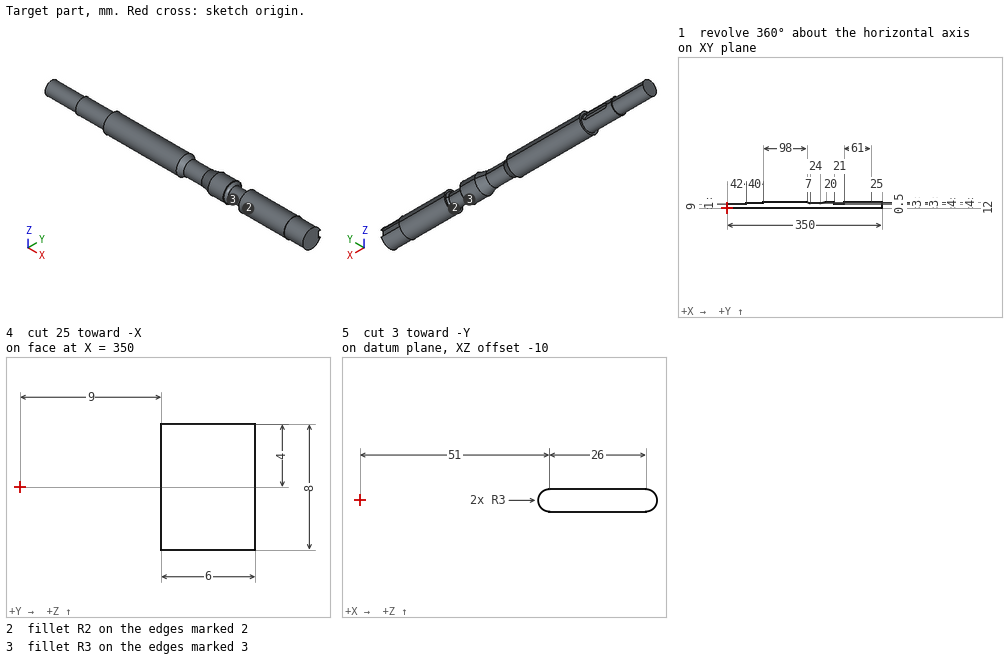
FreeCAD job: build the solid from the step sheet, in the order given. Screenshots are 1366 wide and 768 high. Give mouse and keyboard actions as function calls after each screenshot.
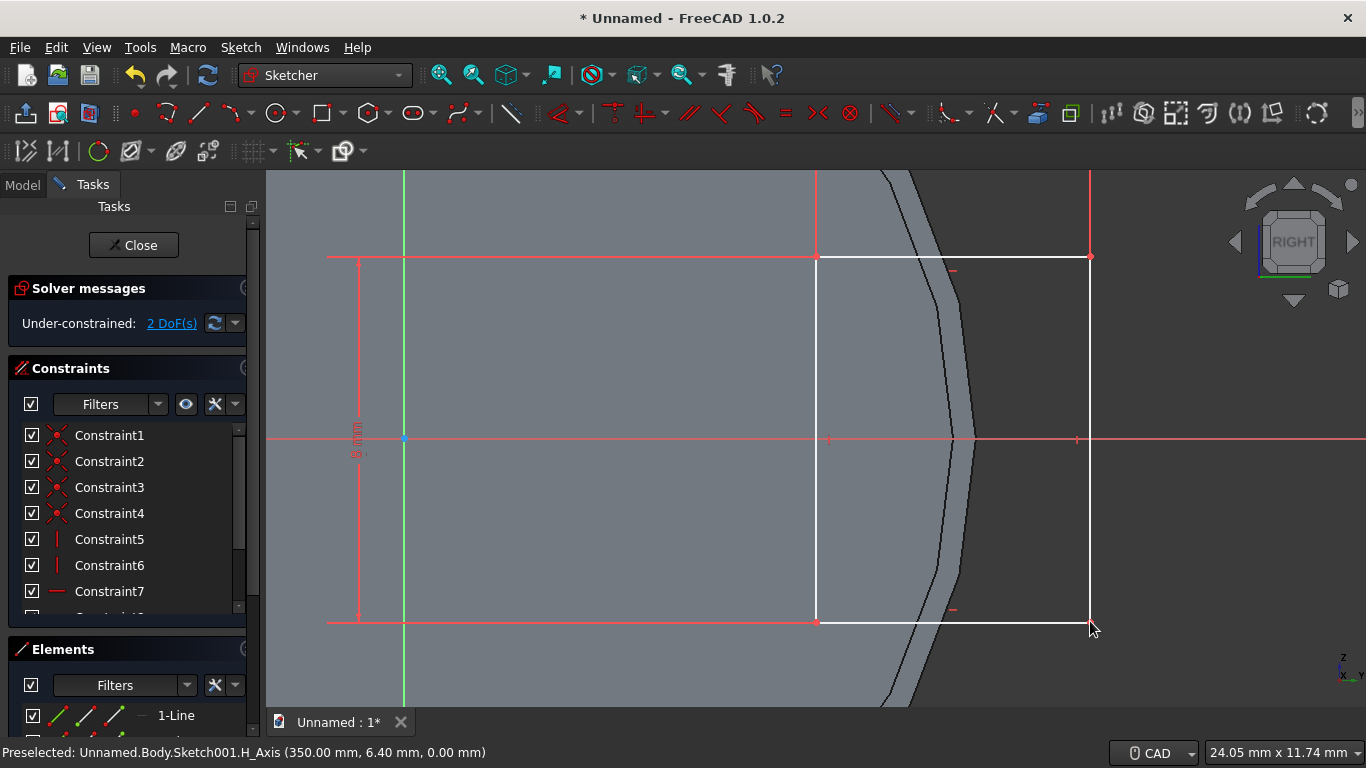
click(558, 114)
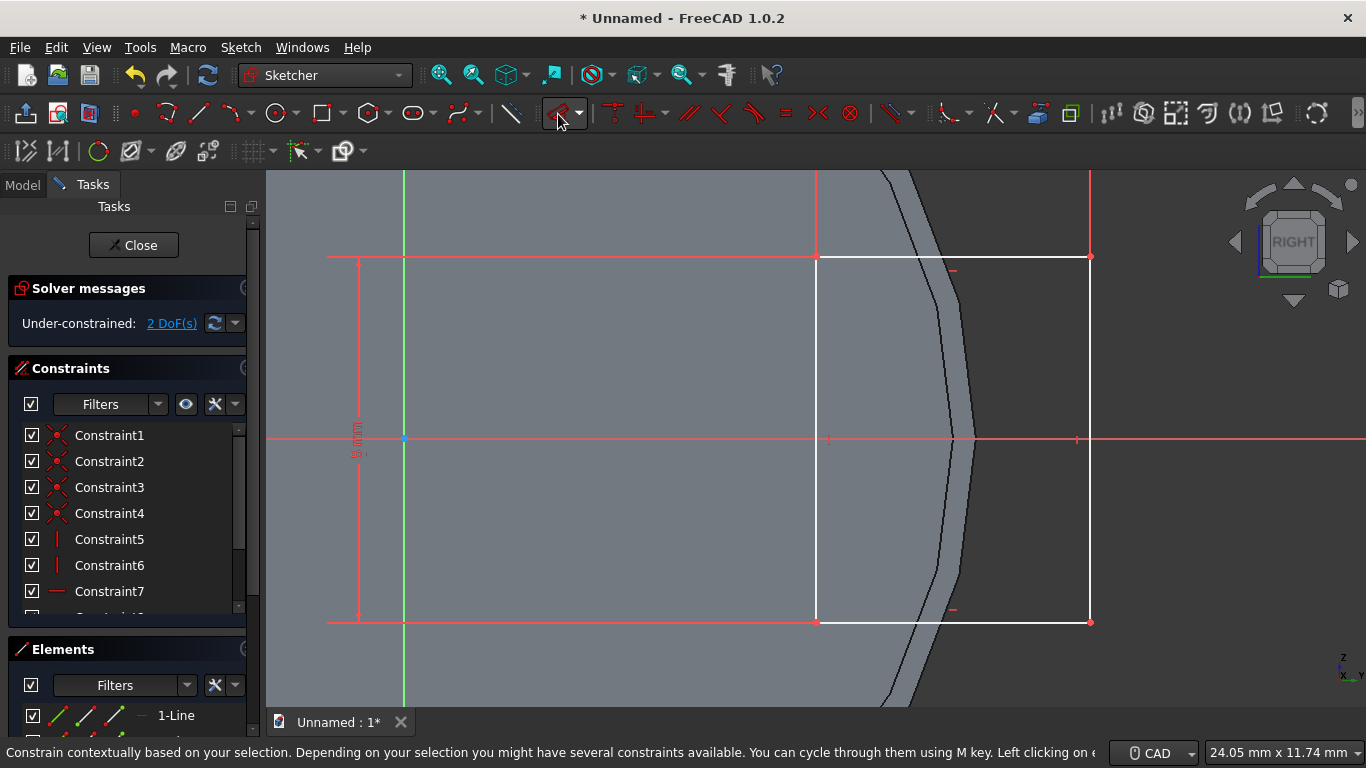
click(816, 257)
click(610, 223)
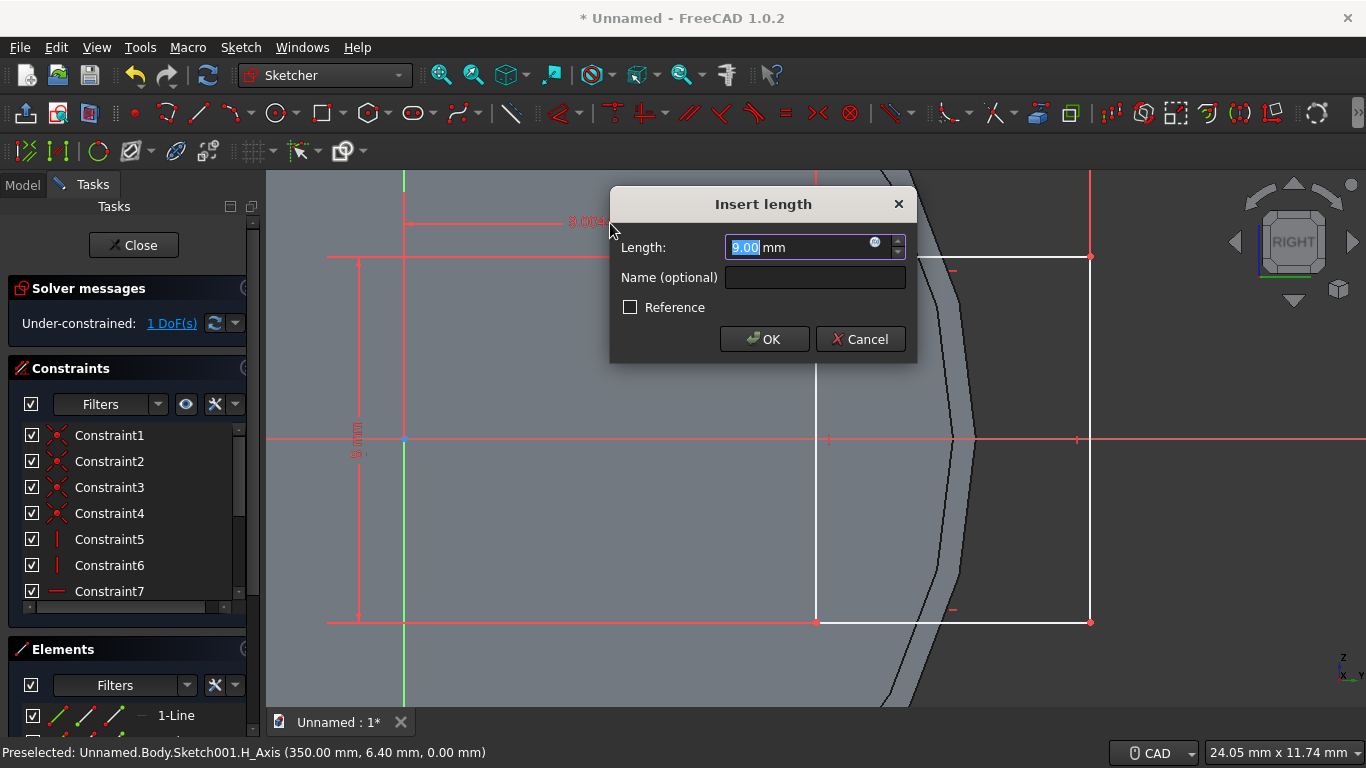
text(9)
key(Return)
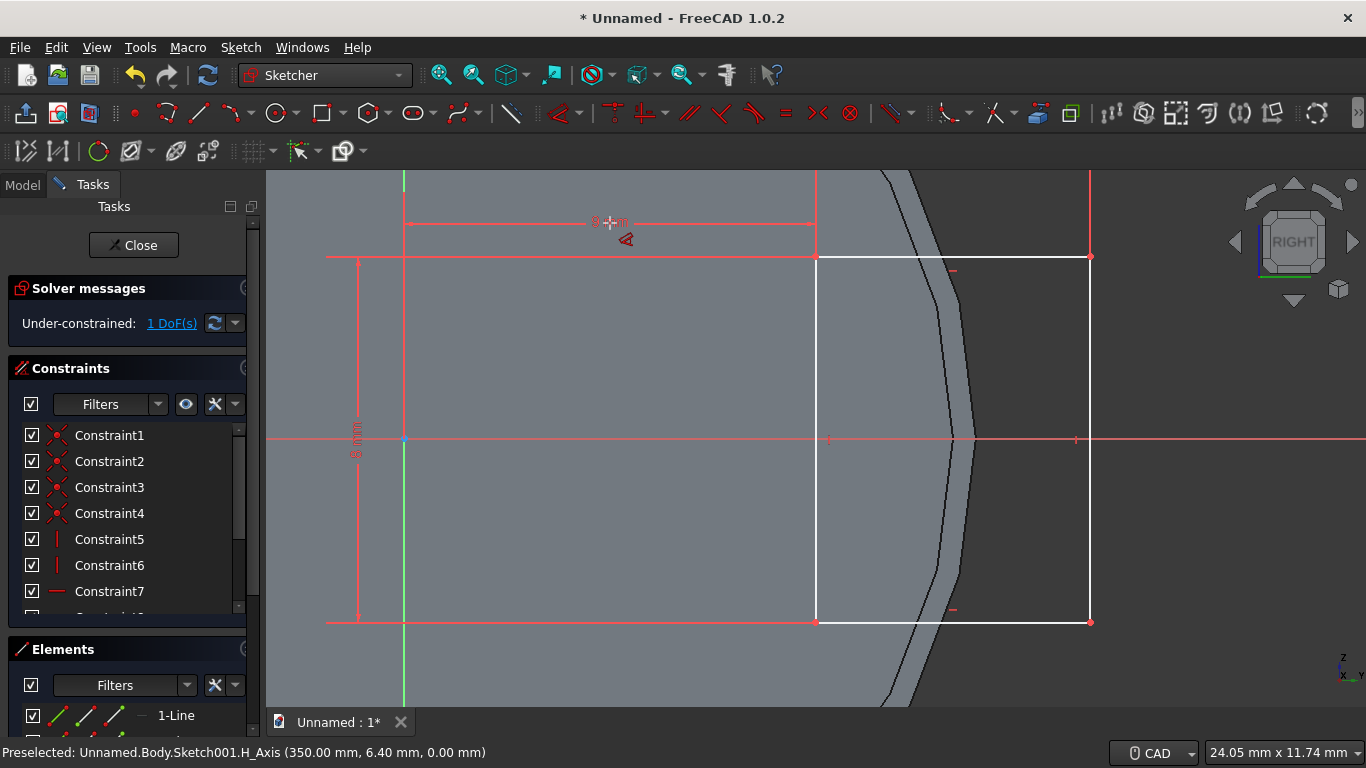
click(816, 257)
click(370, 348)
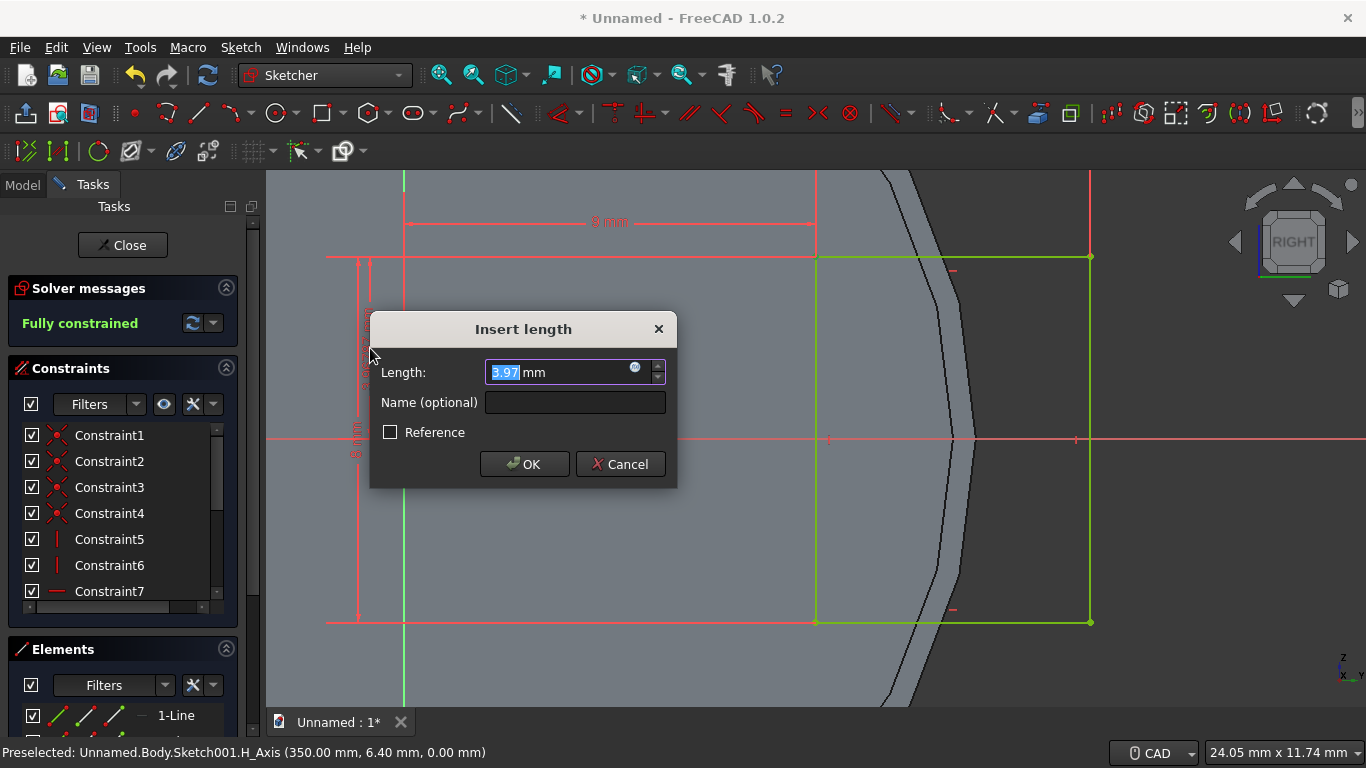
text(4)
key(Return)
key(Escape)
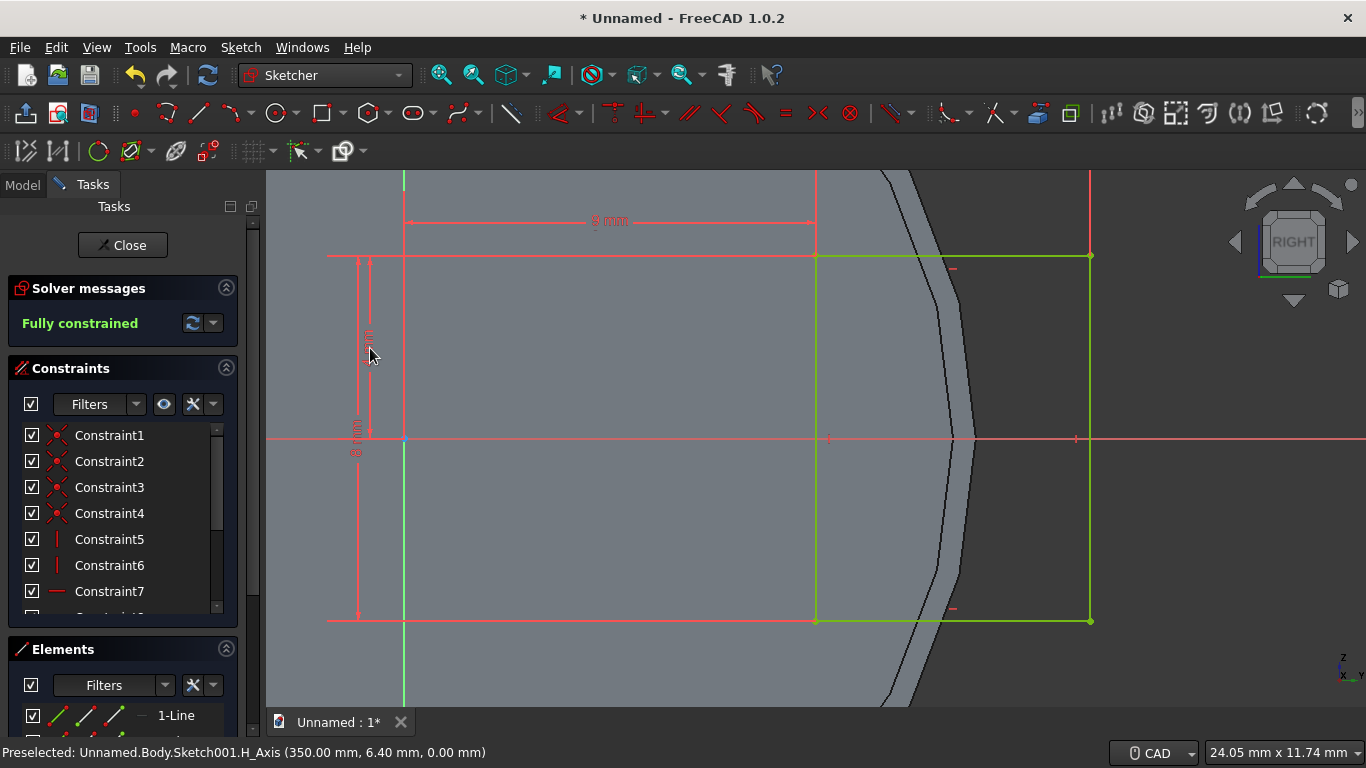
click(123, 245)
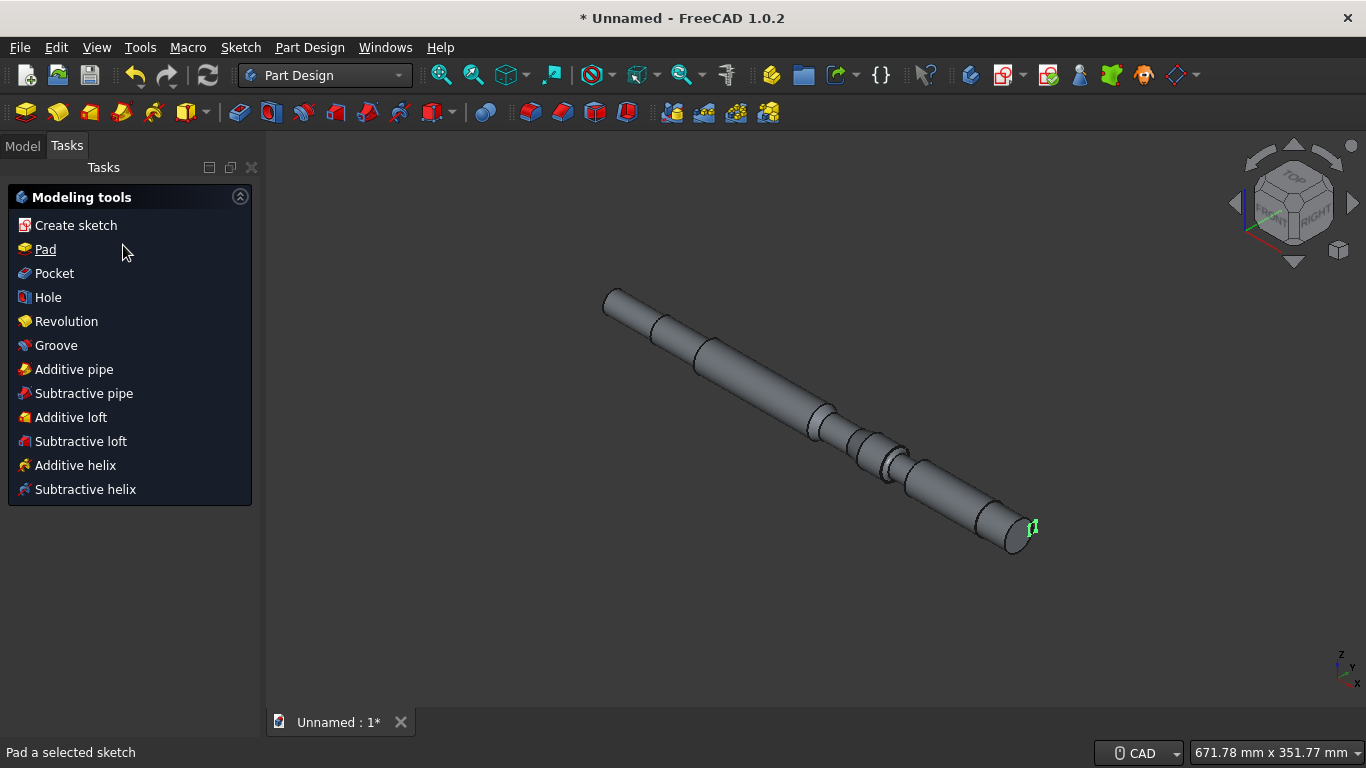
click(240, 112)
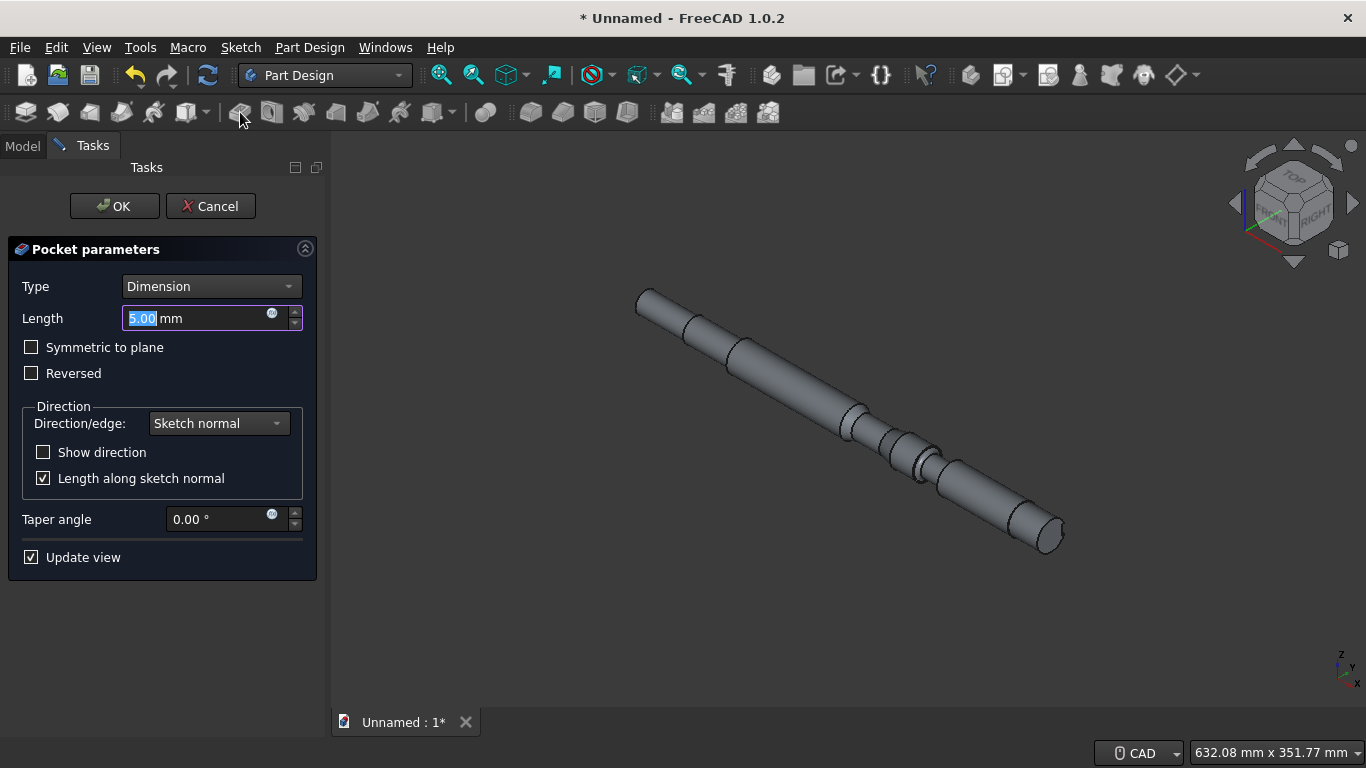
text(25)
key(Tab)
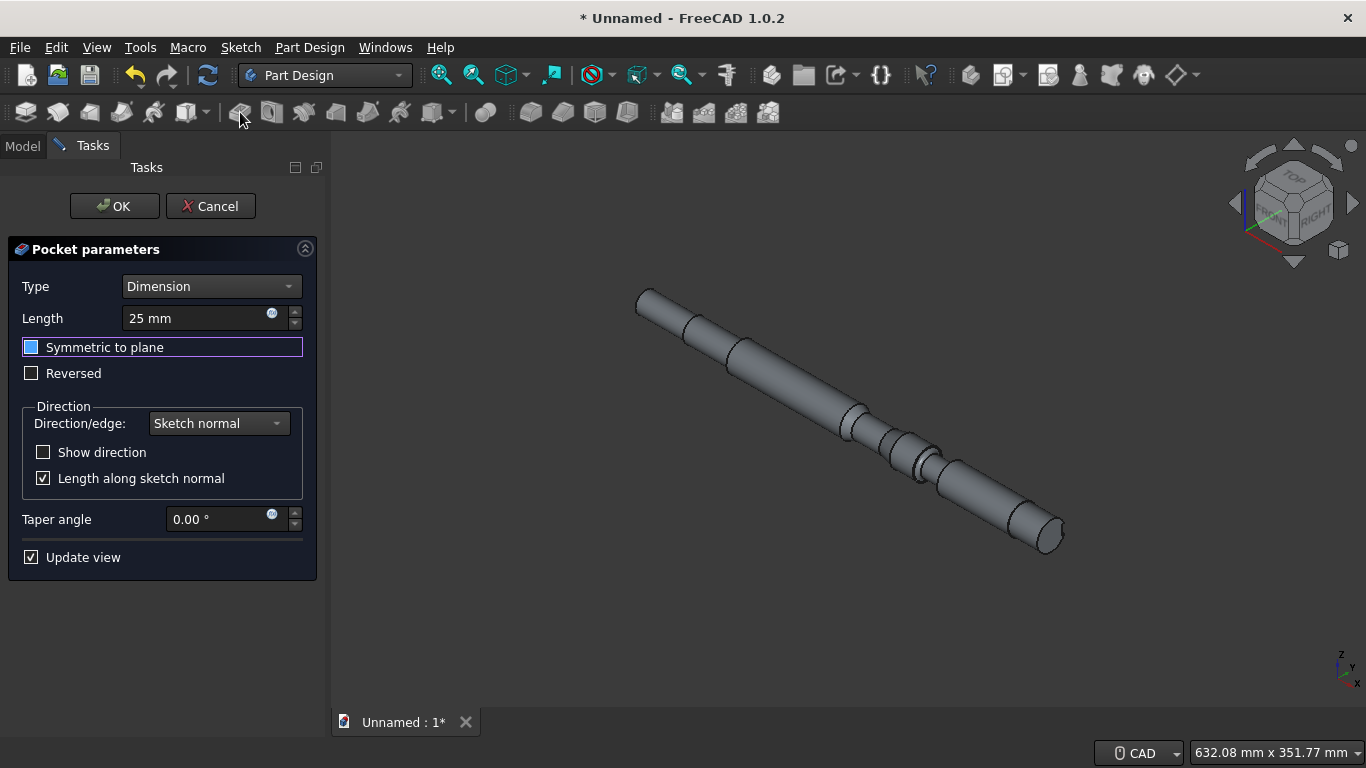
click(115, 206)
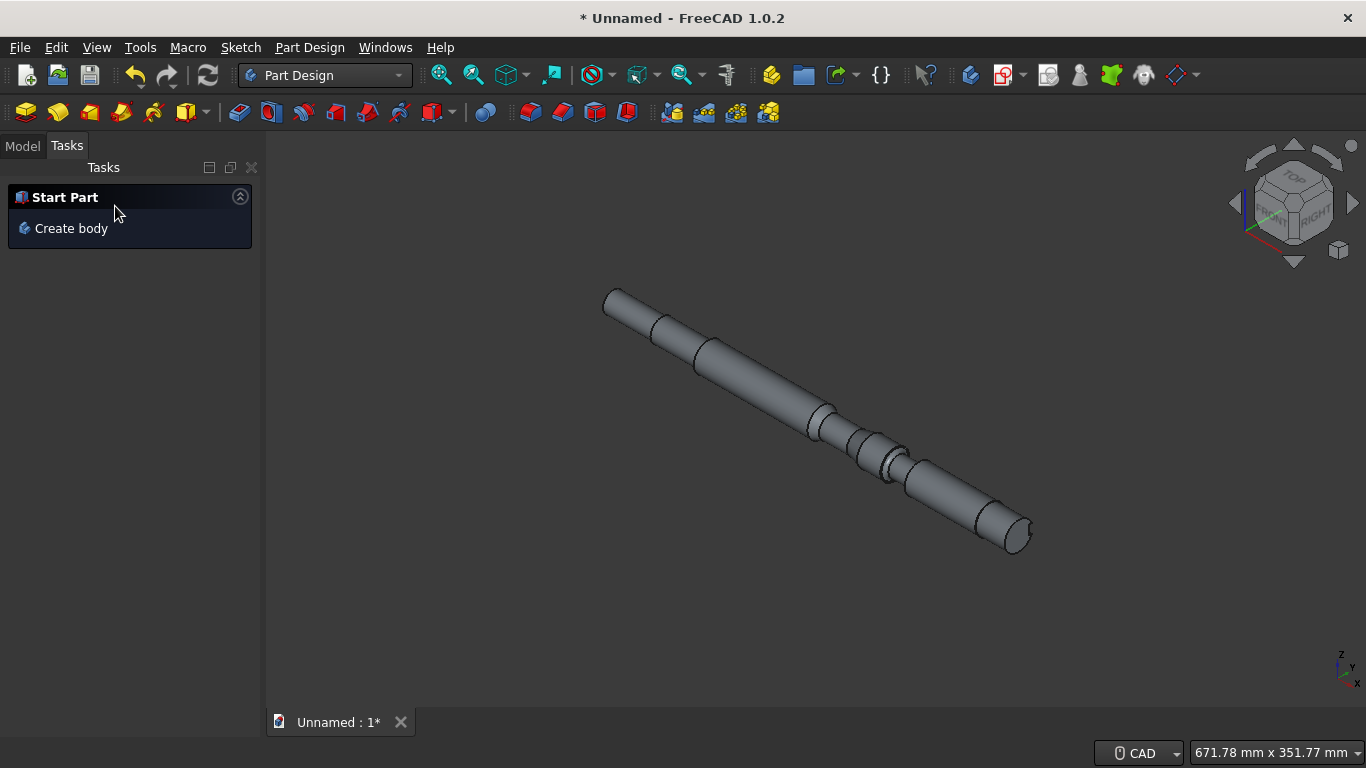
click(23, 145)